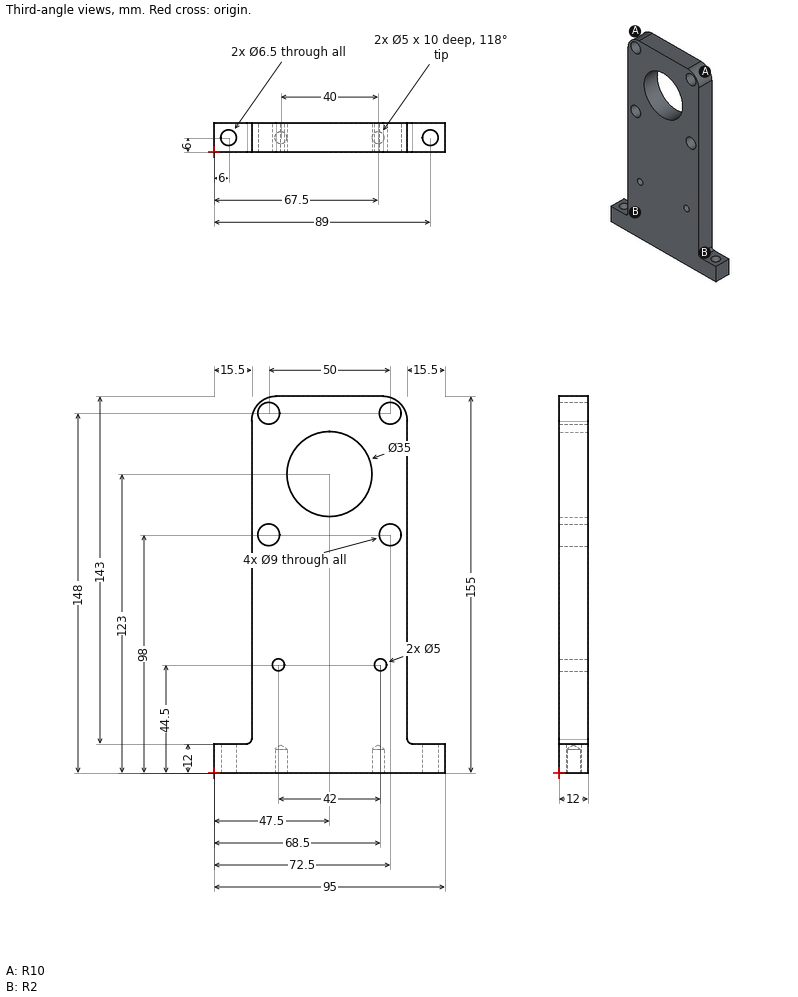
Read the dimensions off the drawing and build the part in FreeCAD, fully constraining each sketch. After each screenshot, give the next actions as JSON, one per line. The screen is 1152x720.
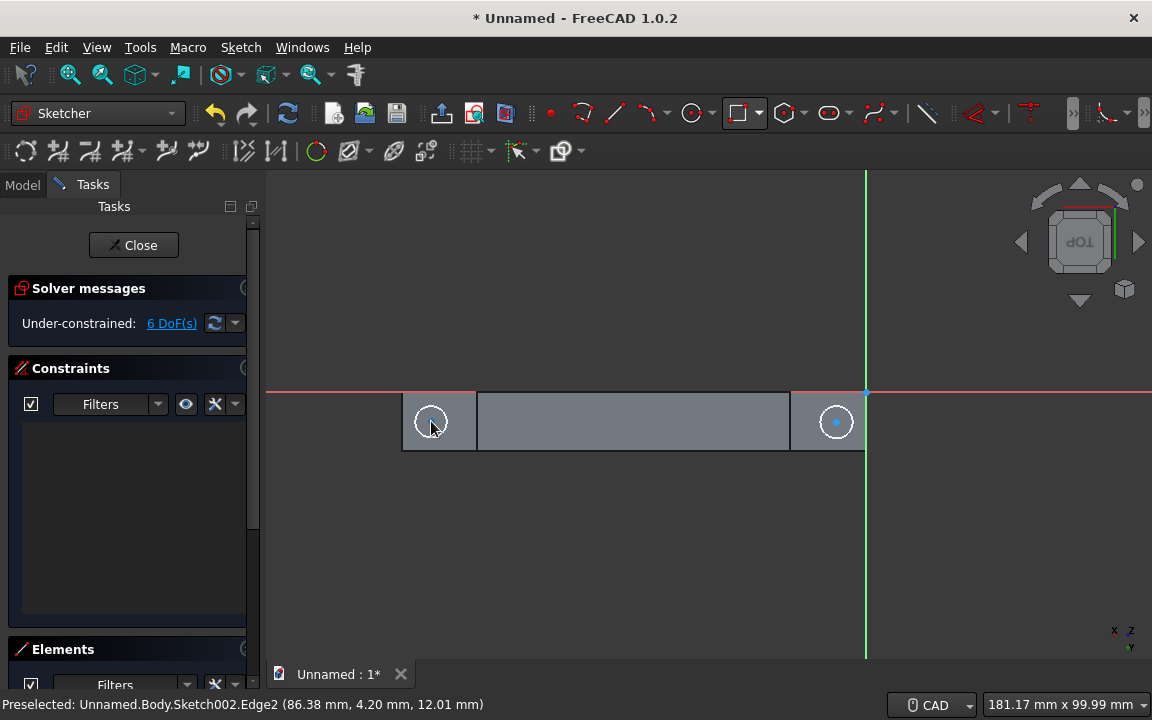
{"action": "left_click", "coordinate": [848, 411]}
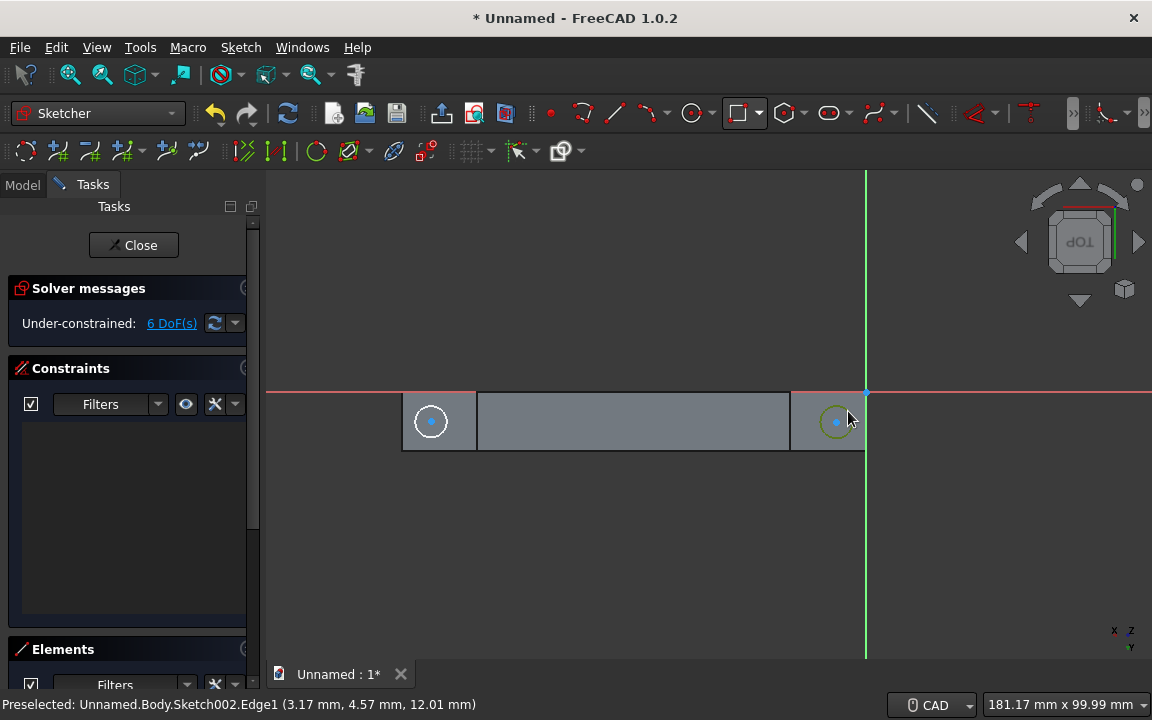
{"action": "left_click", "coordinate": [442, 411]}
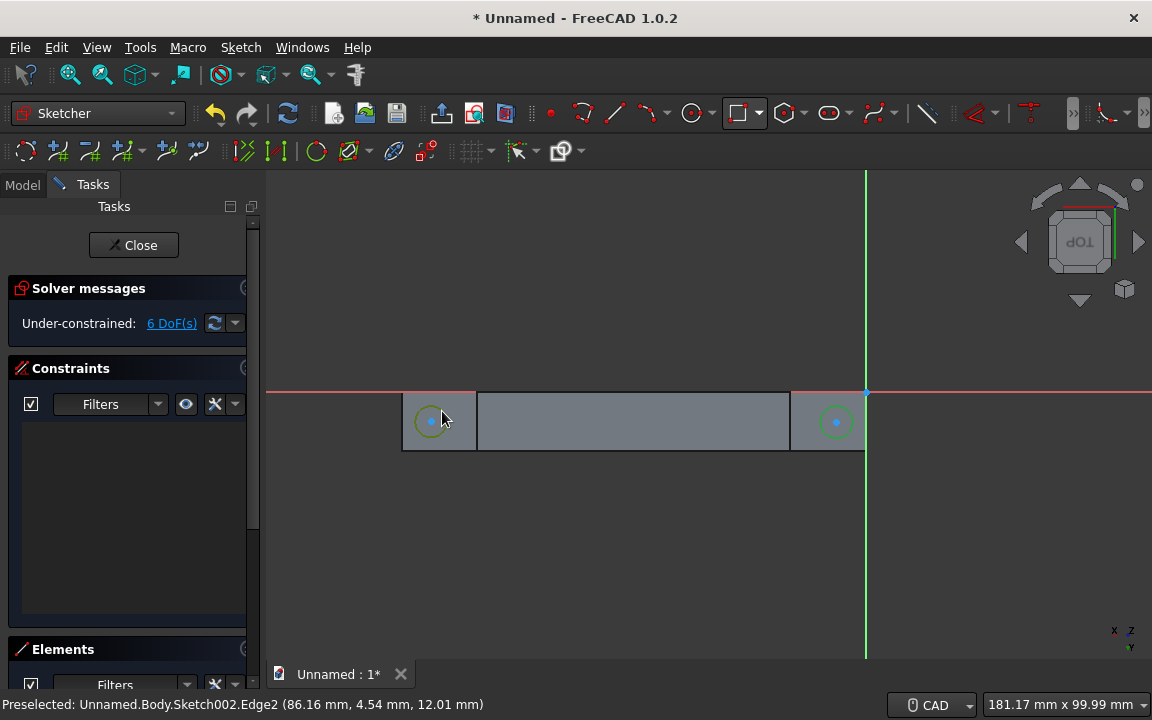
{"action": "key", "text": "e"}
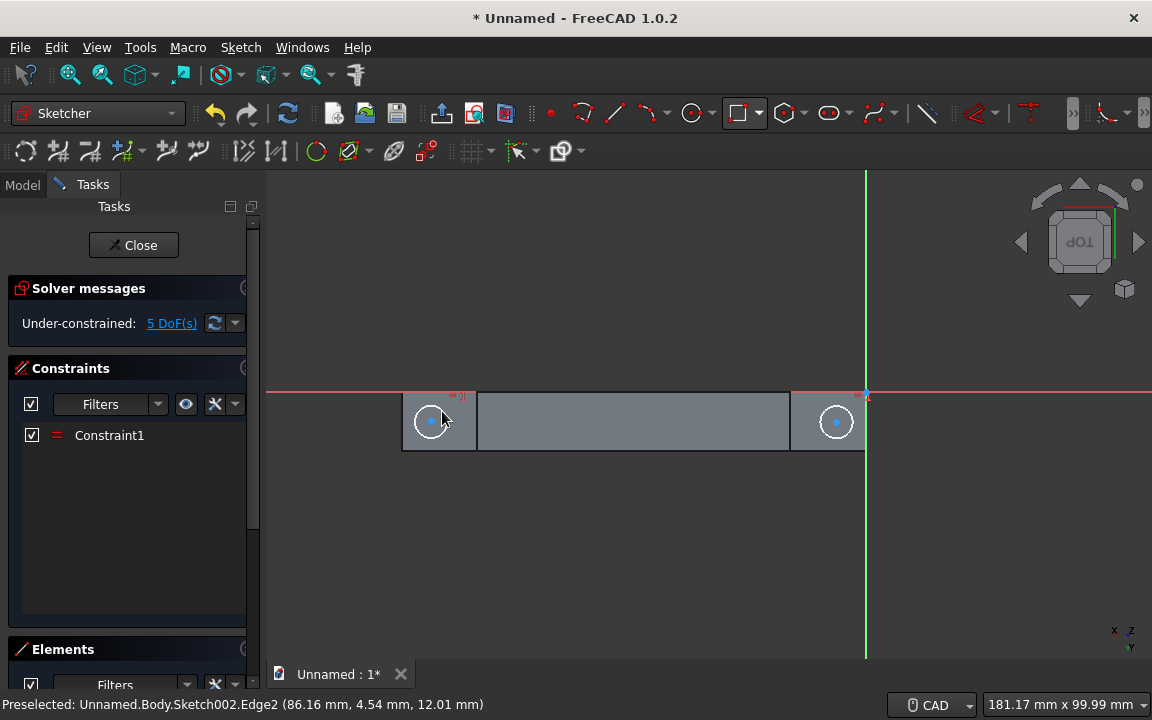
{"action": "left_click", "coordinate": [837, 422]}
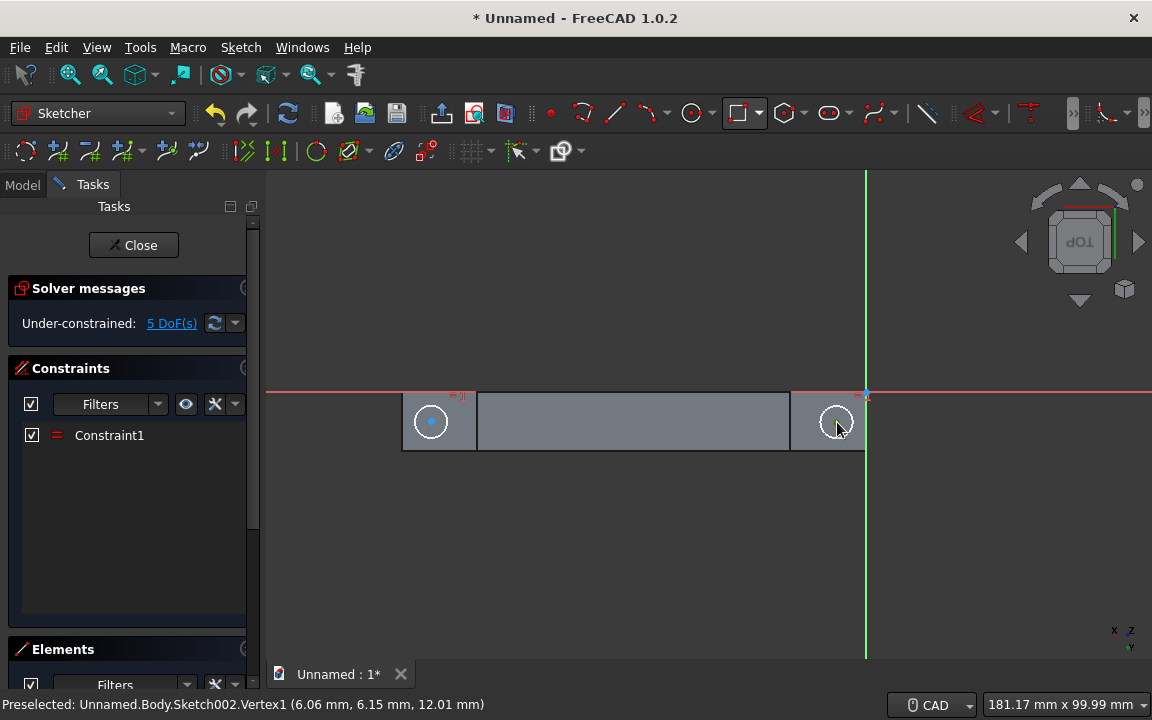
{"action": "left_click", "coordinate": [431, 422]}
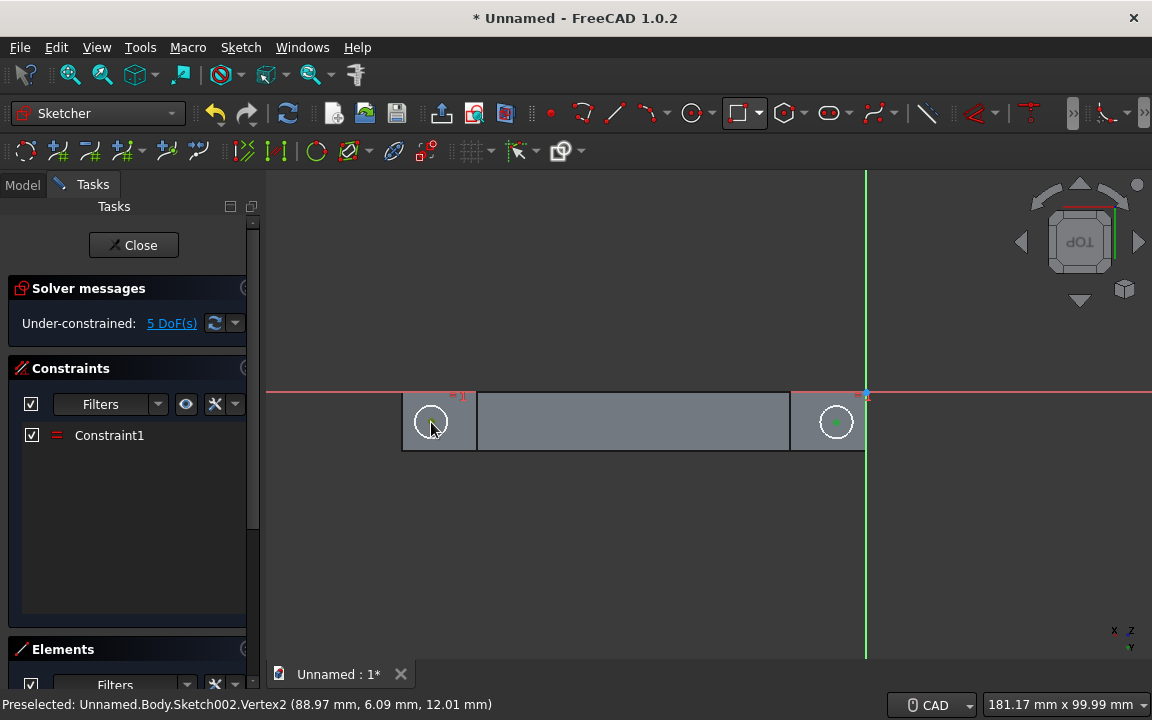
{"action": "key", "text": "h"}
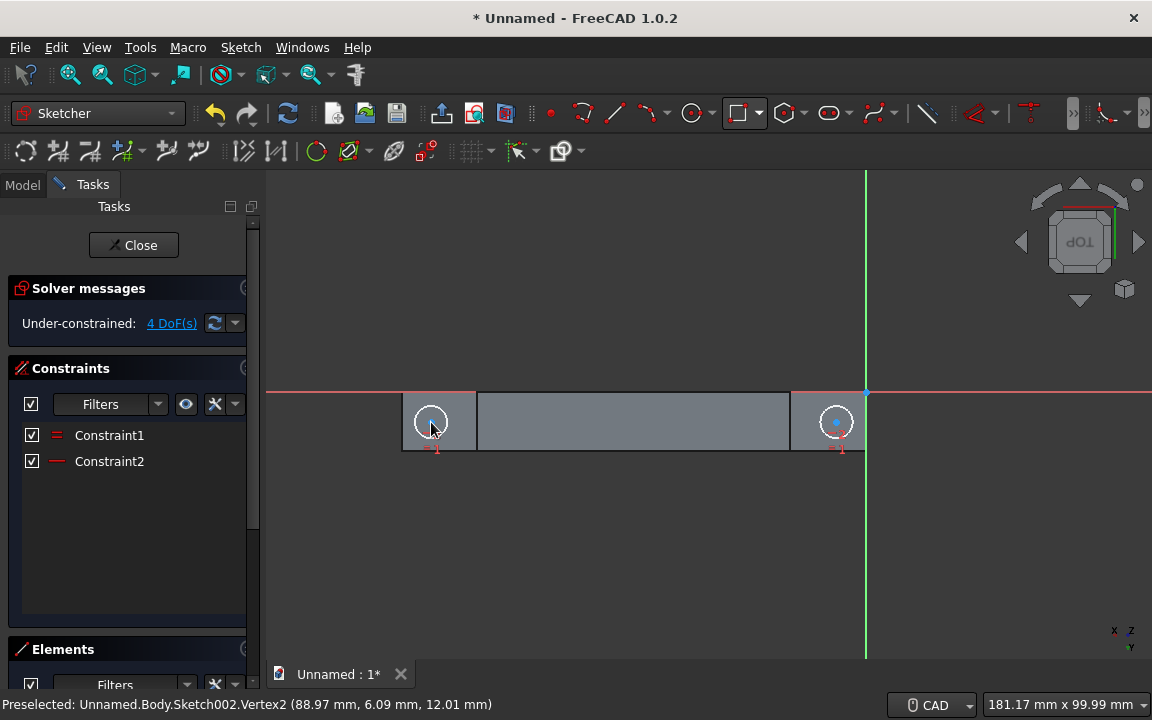
{"action": "left_click", "coordinate": [974, 114]}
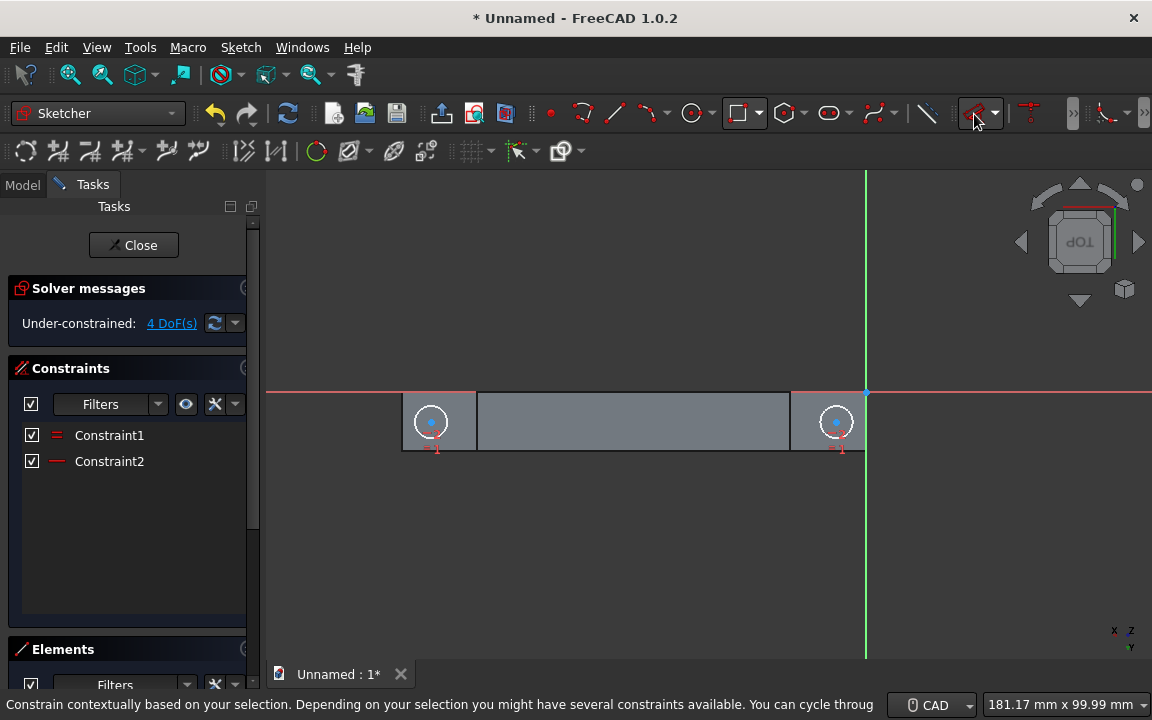
{"action": "scroll", "coordinate": [848, 411], "scroll_direction": "up", "scroll_amount": 2}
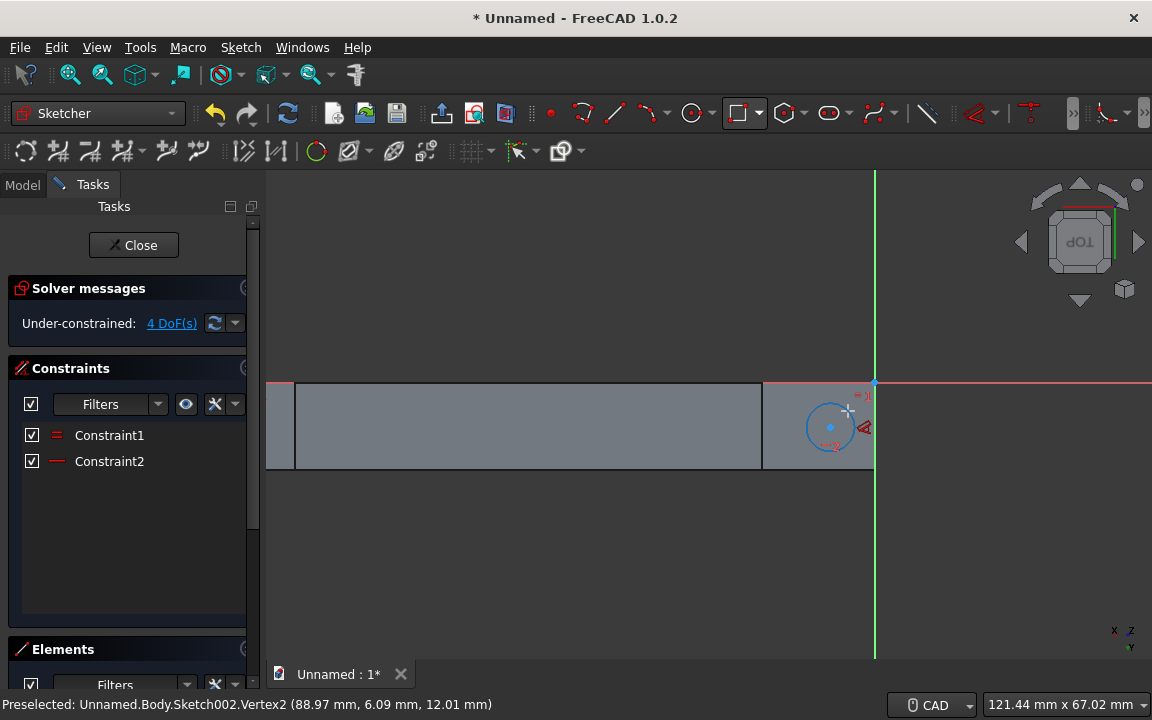
{"action": "left_click", "coordinate": [848, 410]}
{"action": "left_click", "coordinate": [791, 468]}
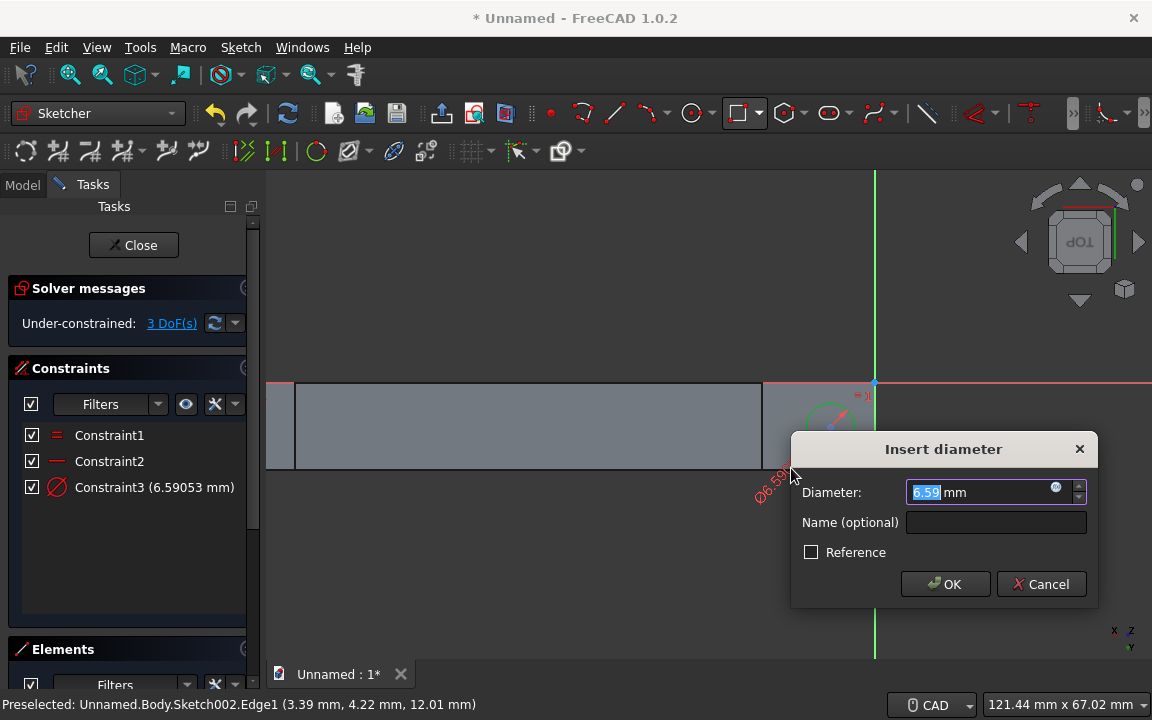
{"action": "type", "text": "6.5"}
{"action": "key", "text": "Return"}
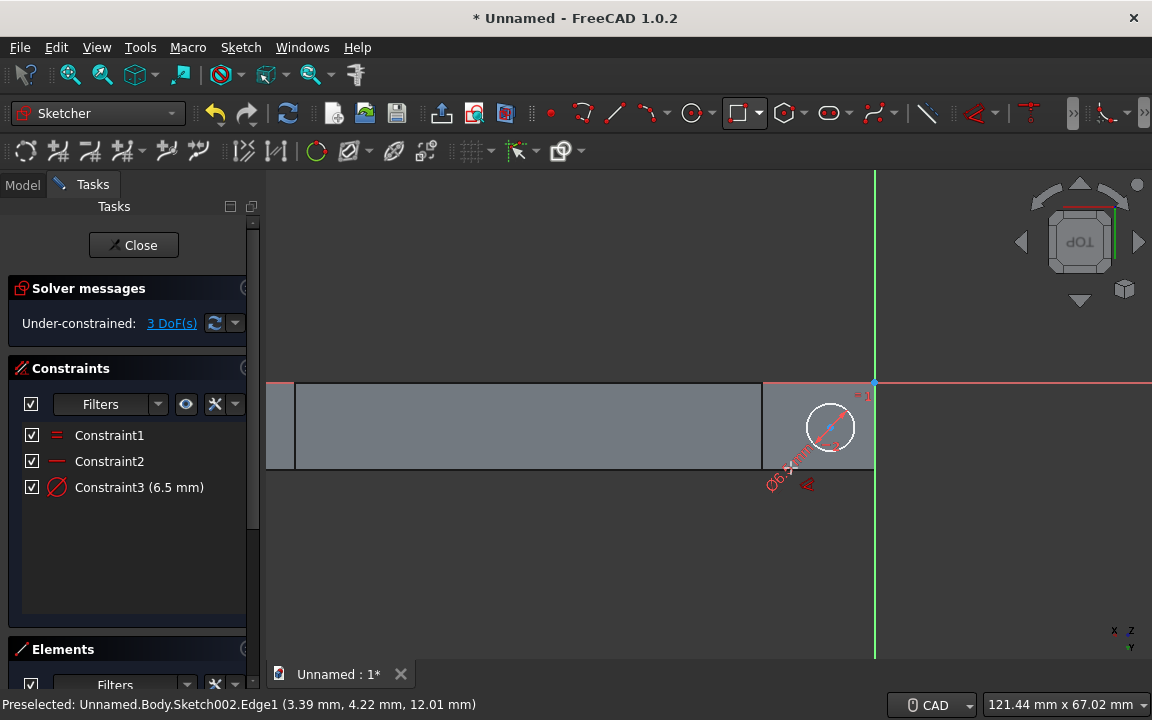
{"action": "left_click", "coordinate": [831, 427]}
{"action": "left_click", "coordinate": [853, 349]}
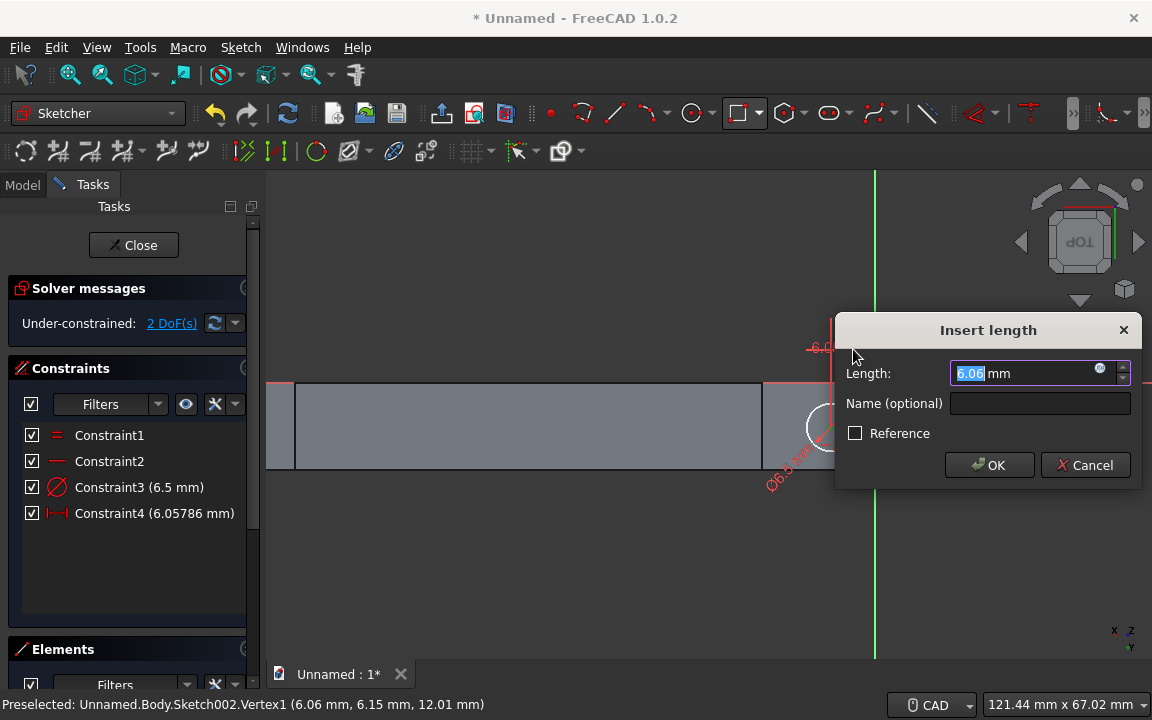
{"action": "type", "text": "6"}
{"action": "key", "text": "Return"}